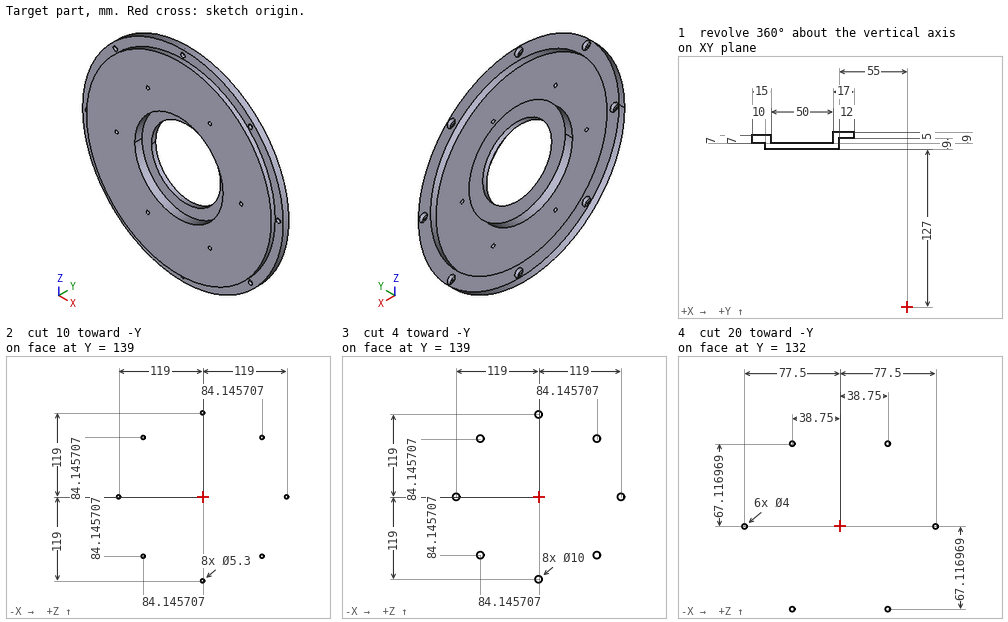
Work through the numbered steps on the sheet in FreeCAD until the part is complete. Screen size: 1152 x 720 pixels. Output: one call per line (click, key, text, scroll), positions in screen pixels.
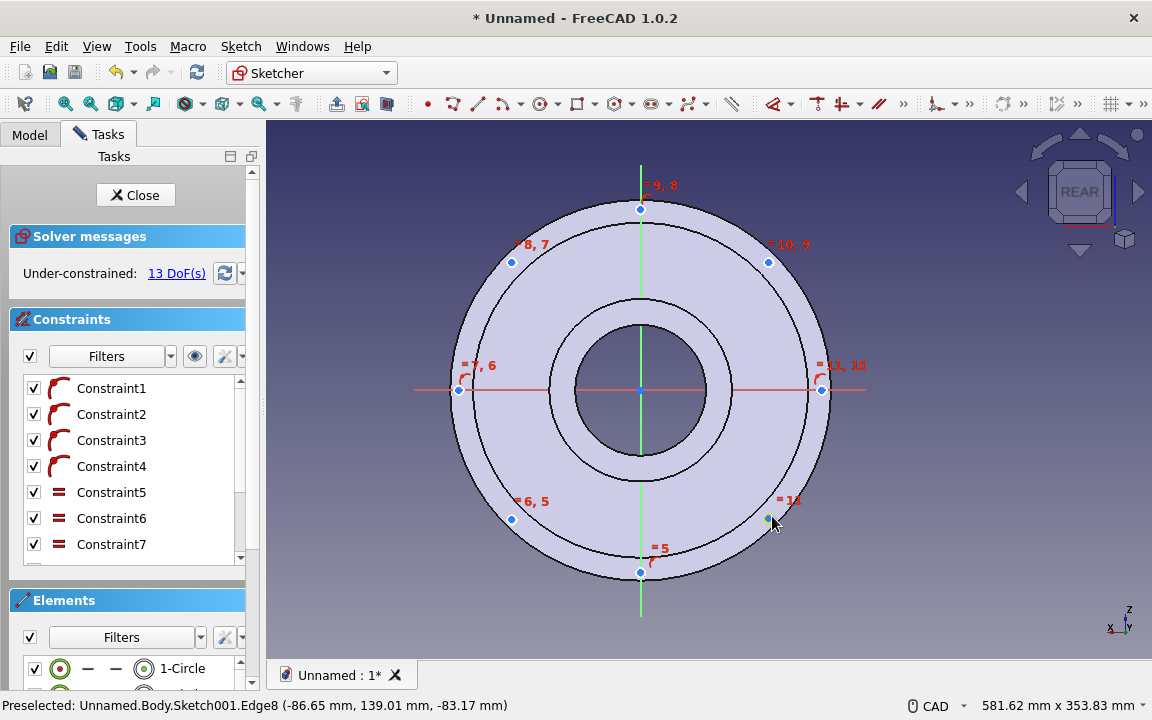
click(512, 520)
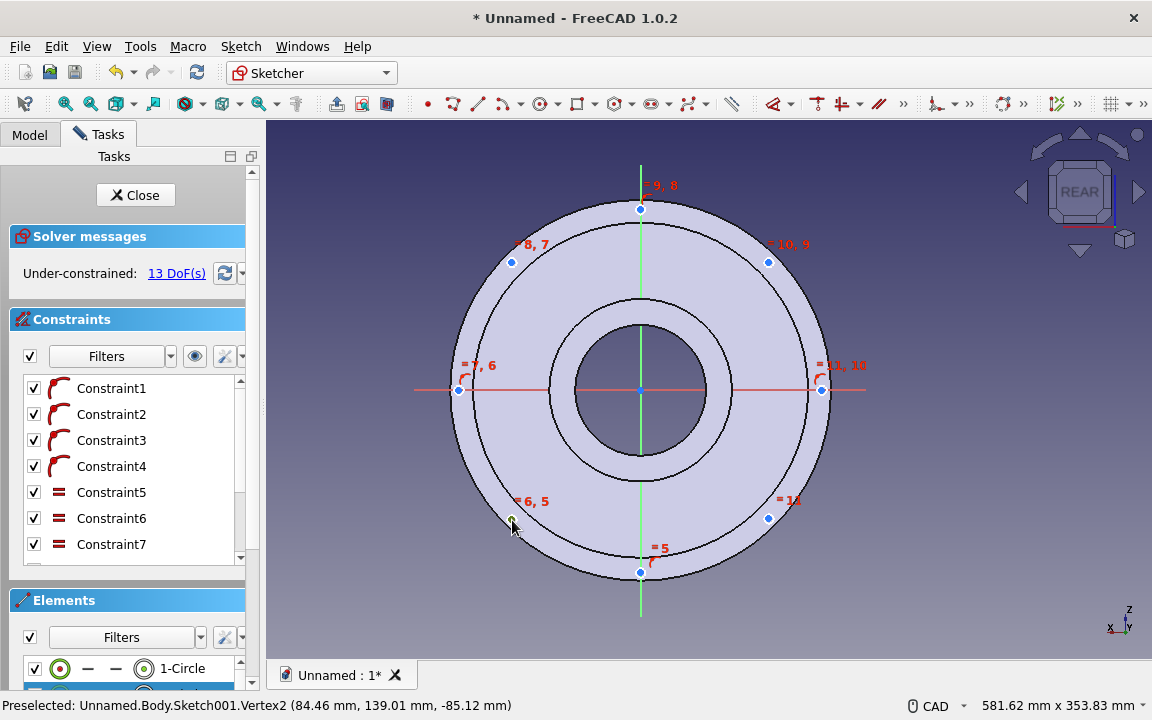
click(512, 263)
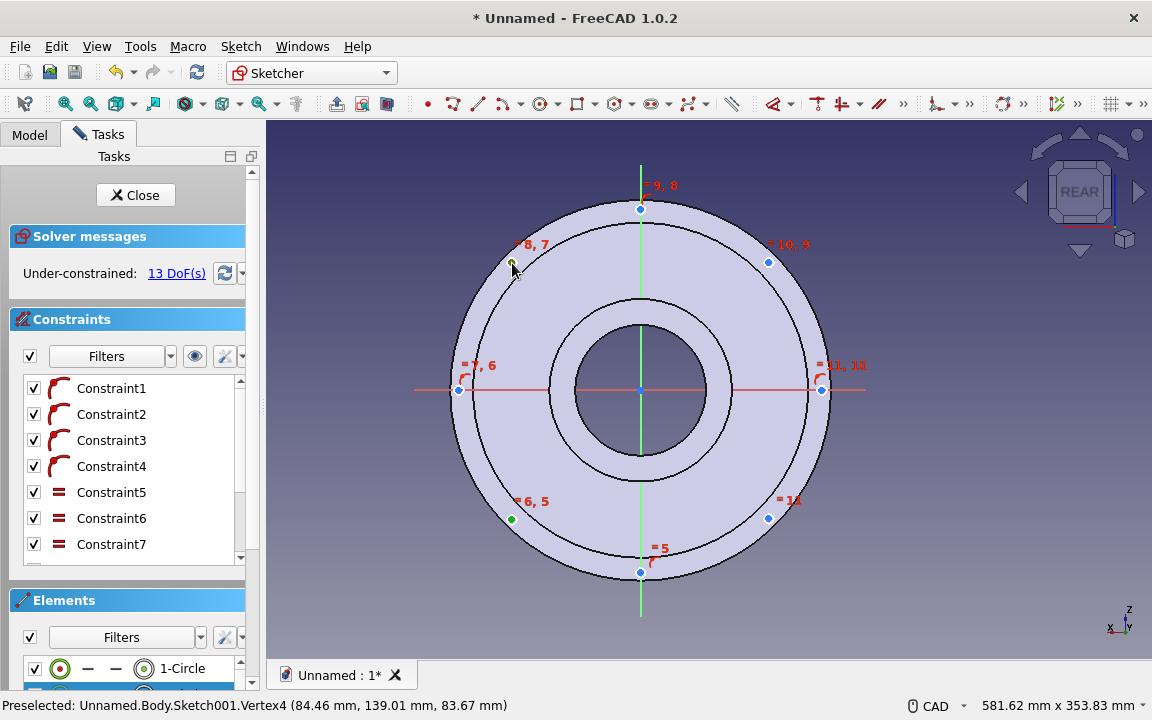
key(v)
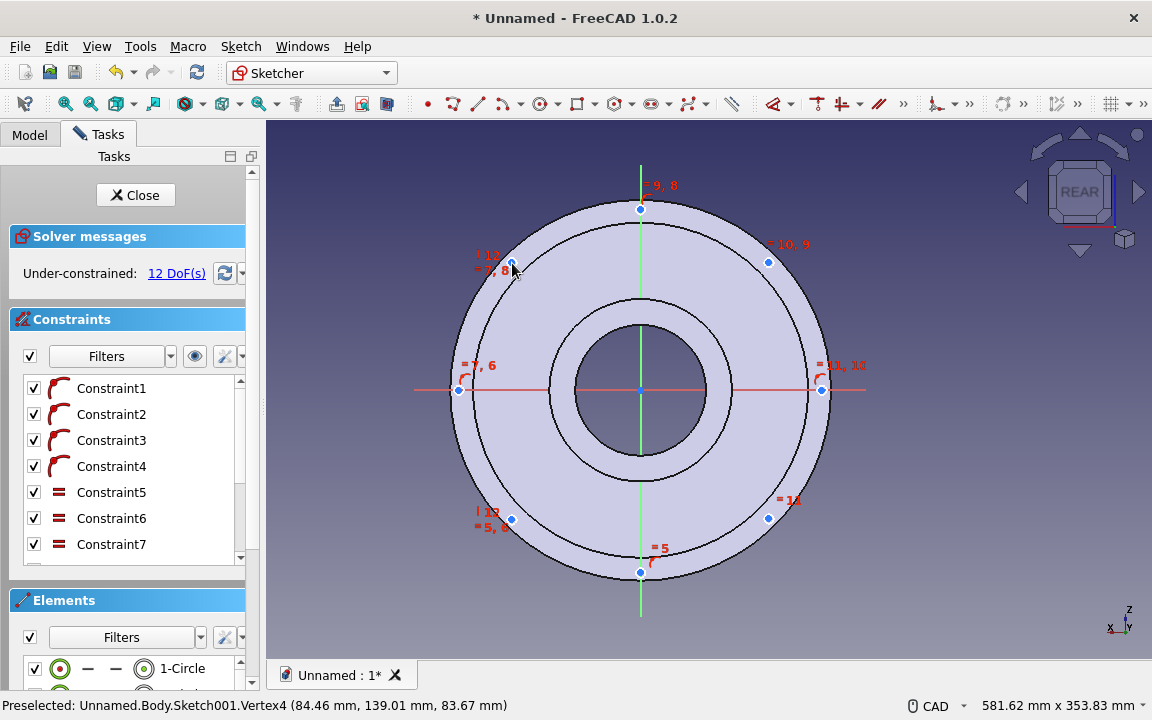
click(512, 263)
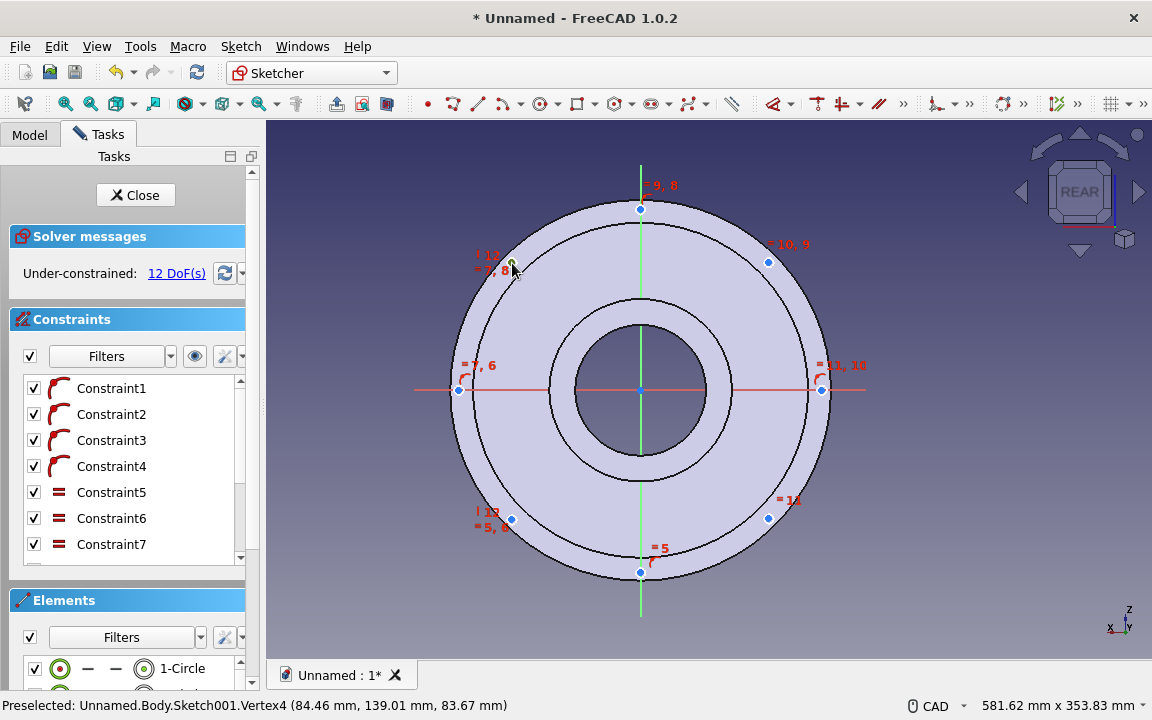
click(769, 263)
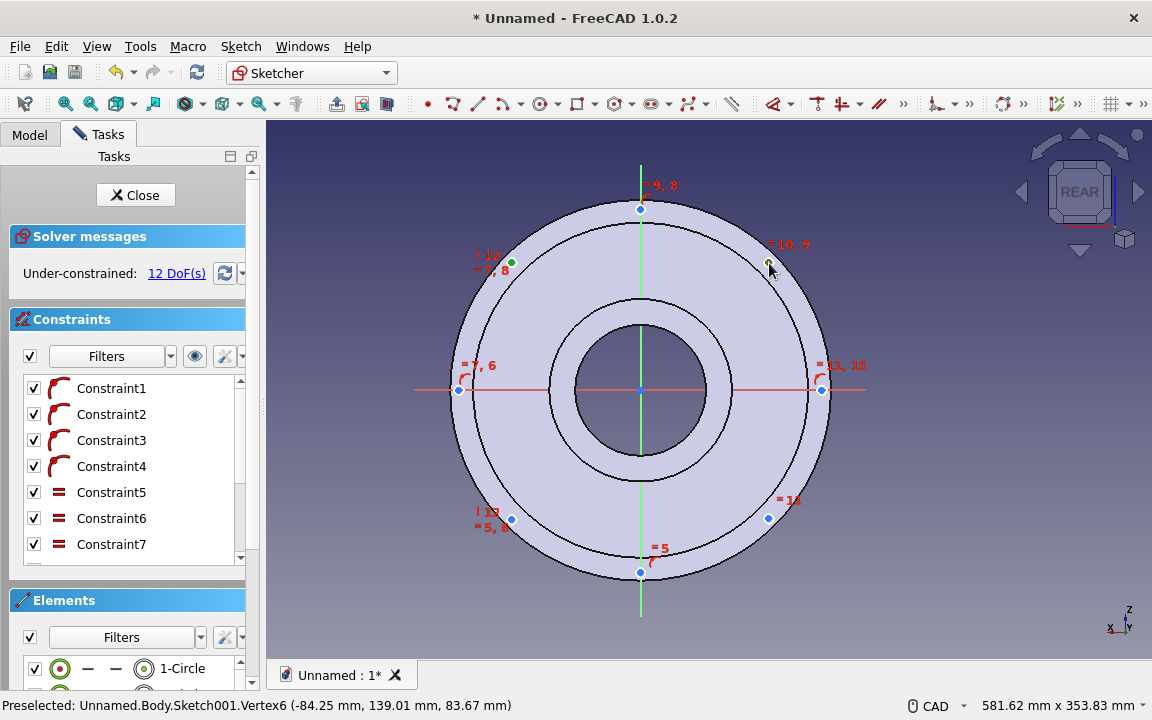
click(860, 104)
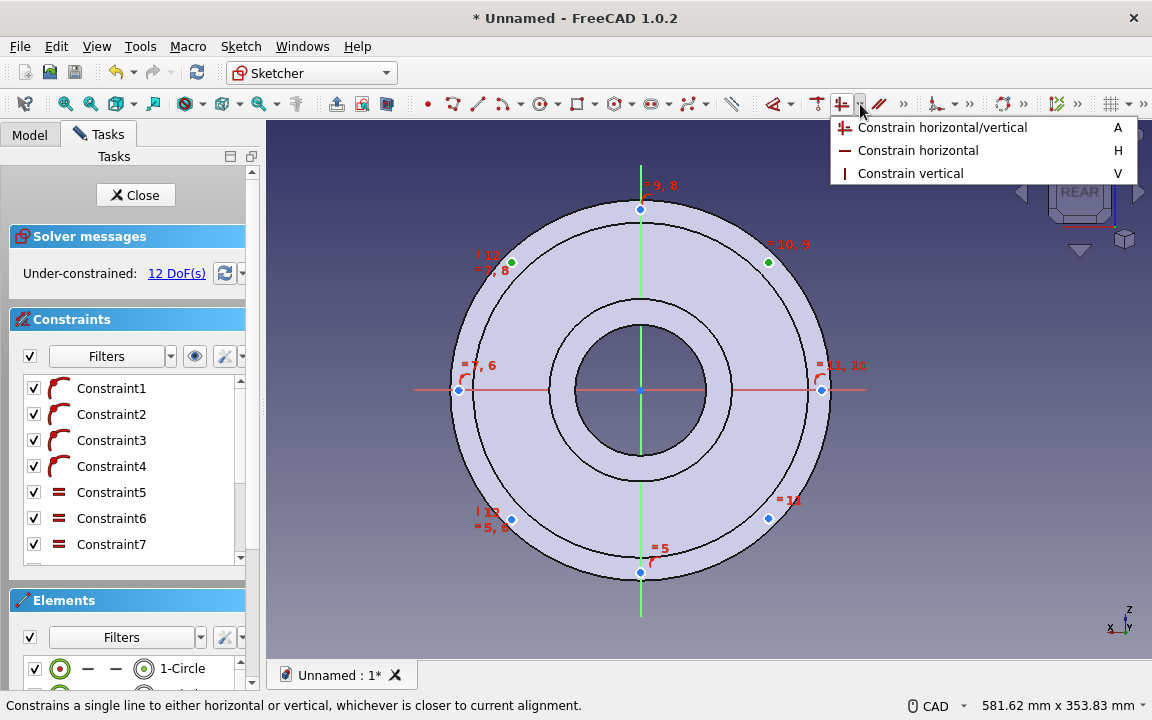
click(984, 150)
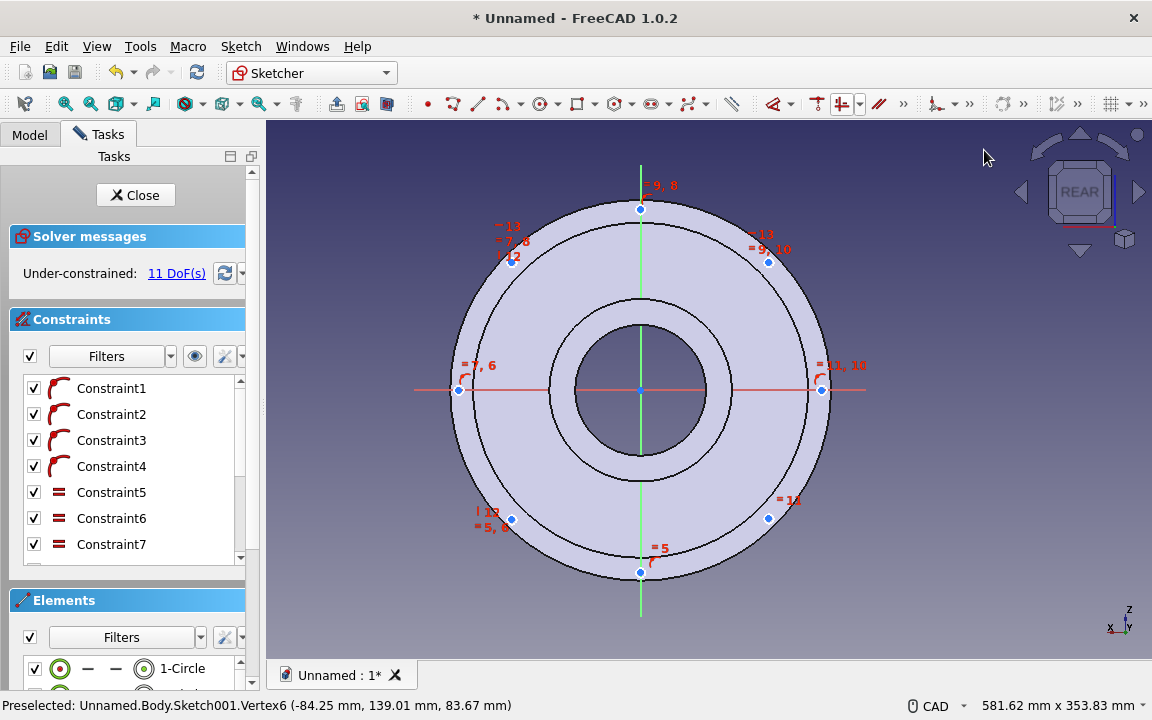
click(769, 263)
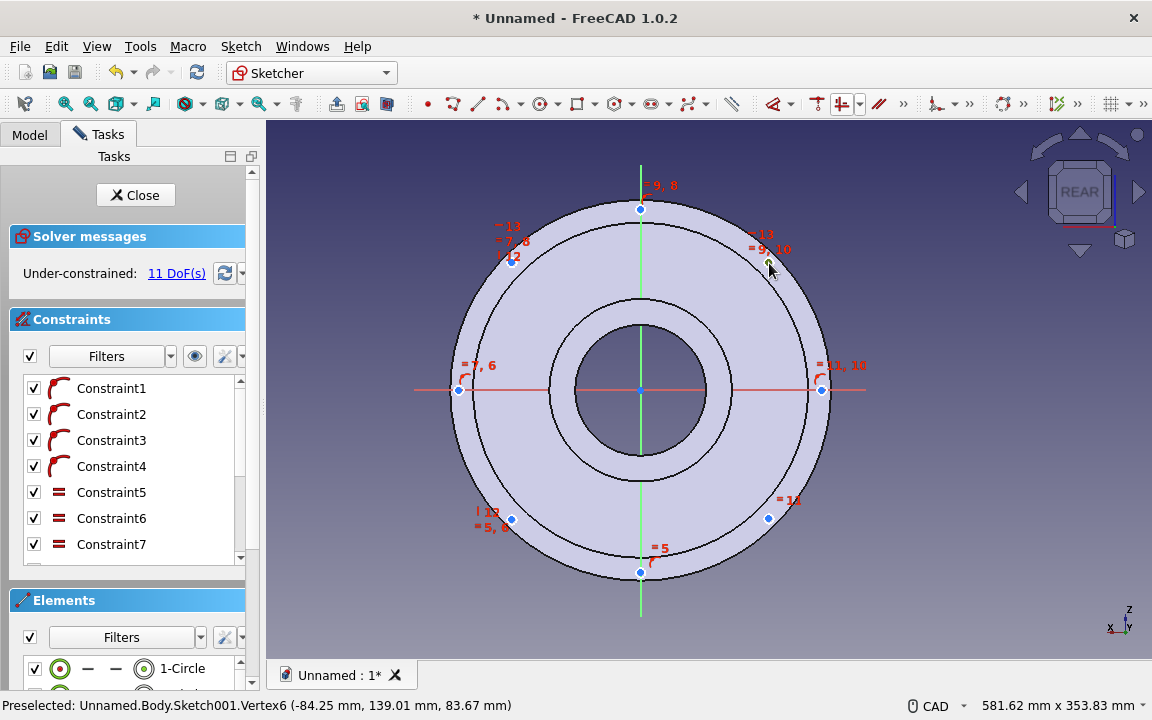
click(769, 519)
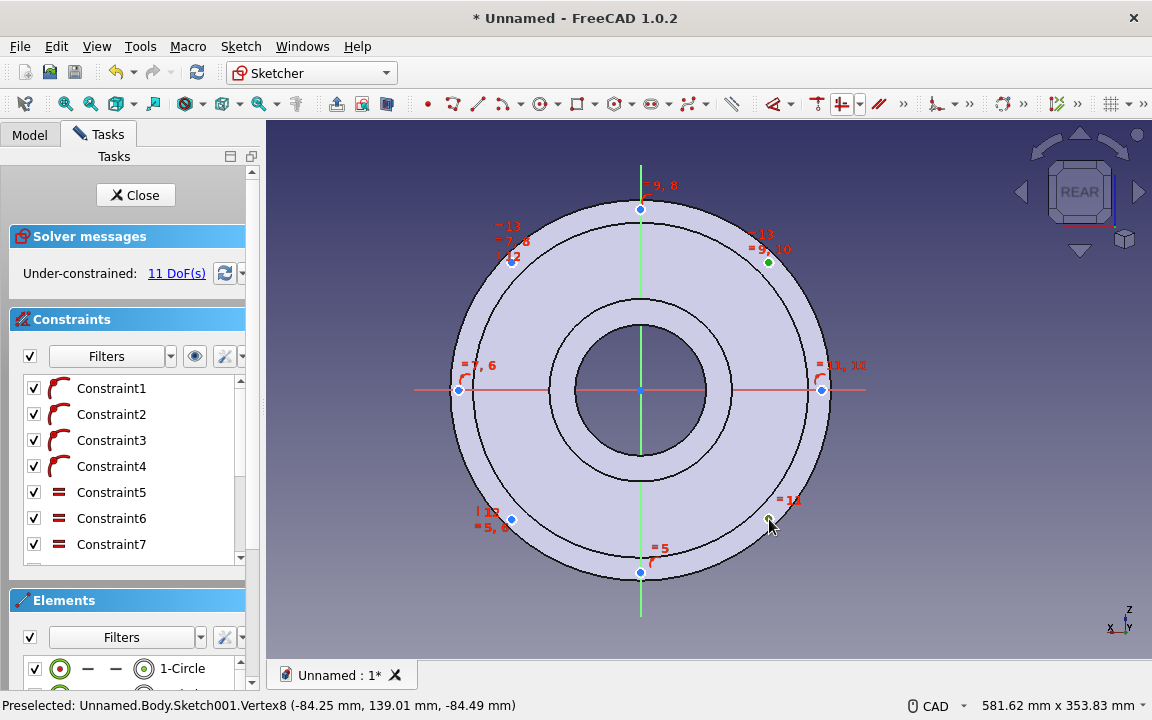
key(v)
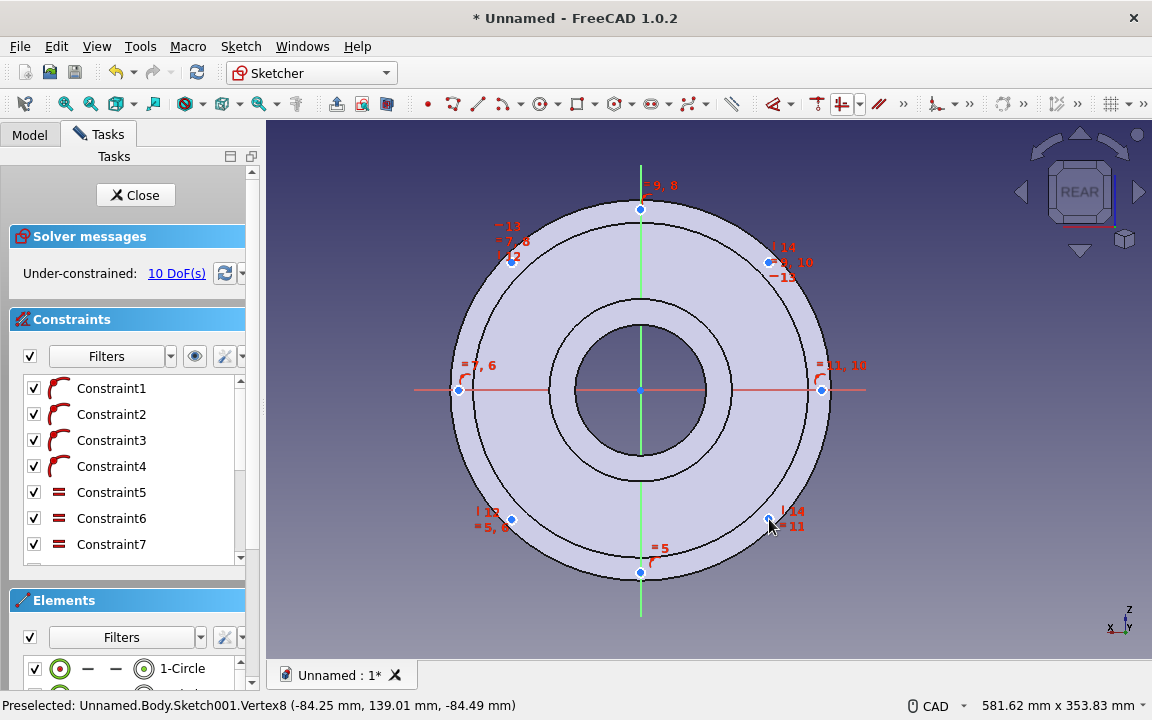
click(512, 520)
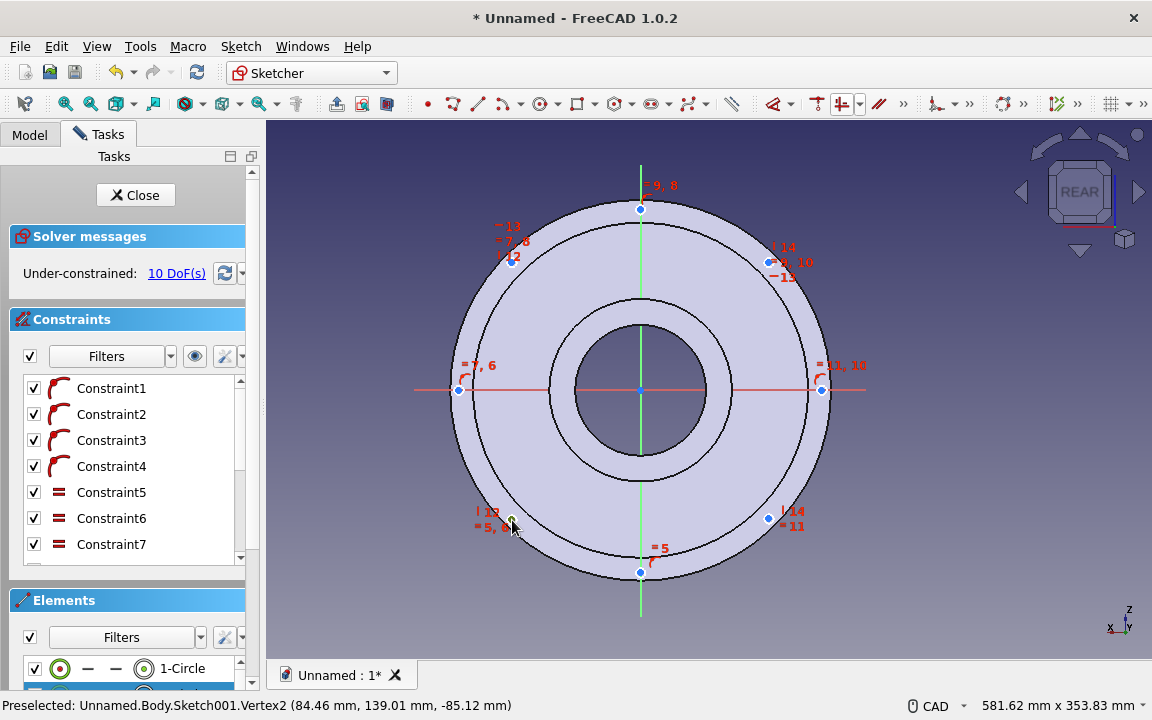
click(769, 519)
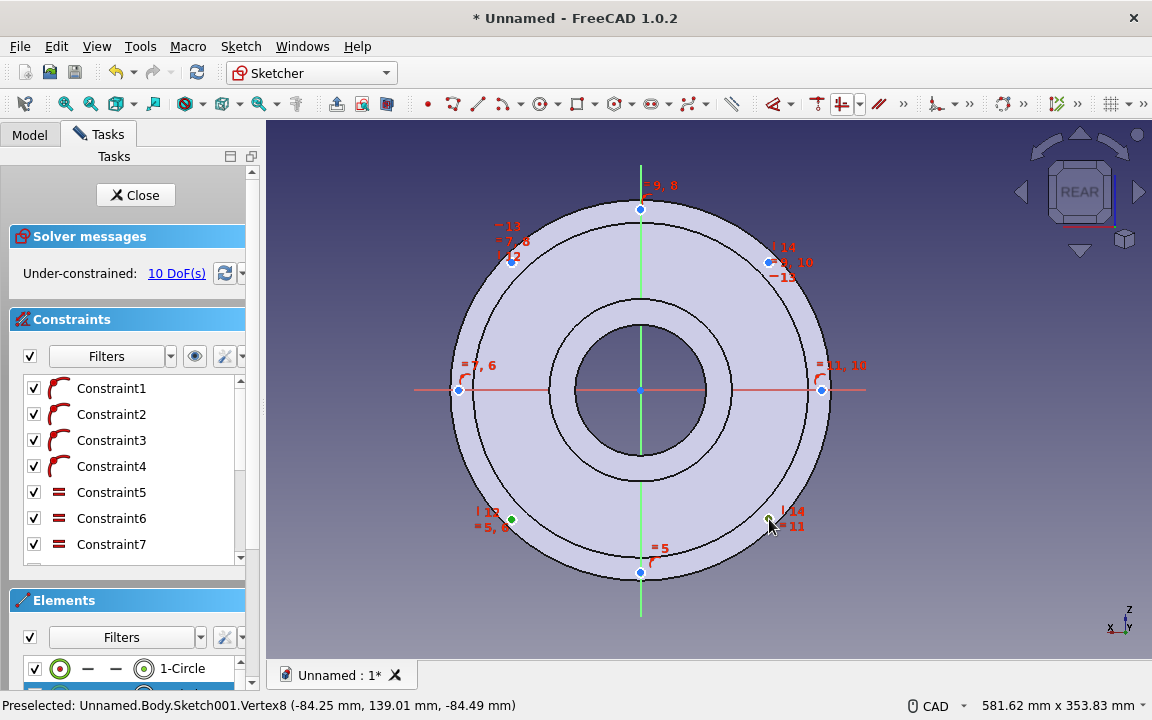
click(860, 104)